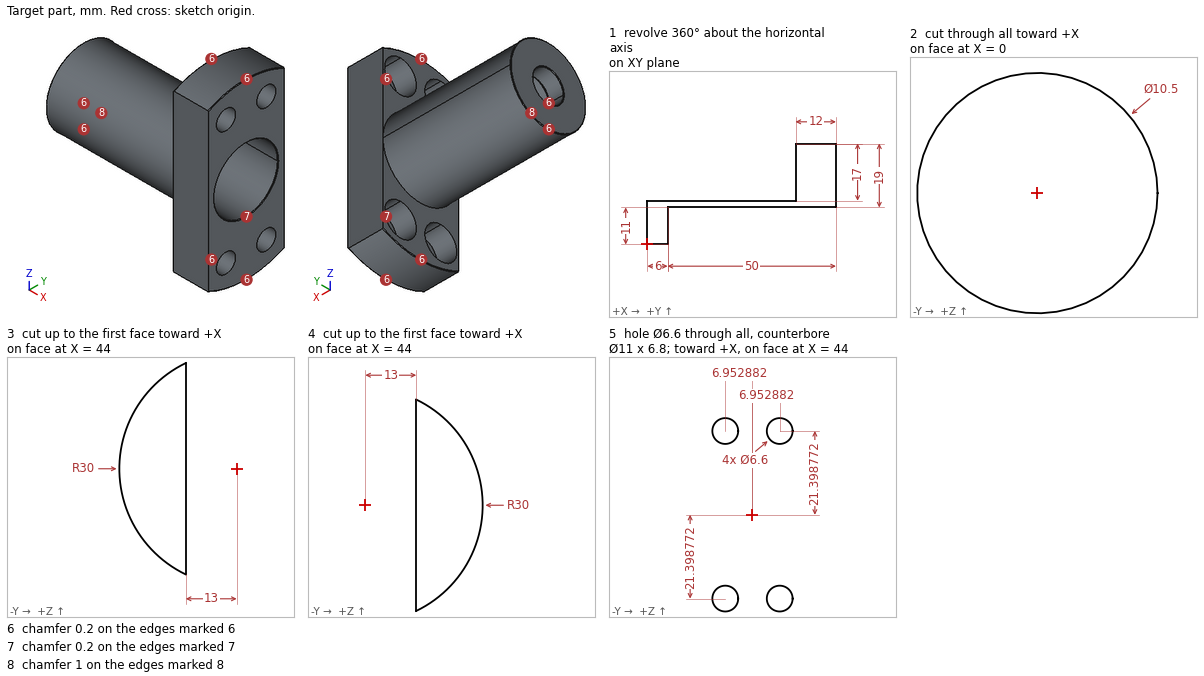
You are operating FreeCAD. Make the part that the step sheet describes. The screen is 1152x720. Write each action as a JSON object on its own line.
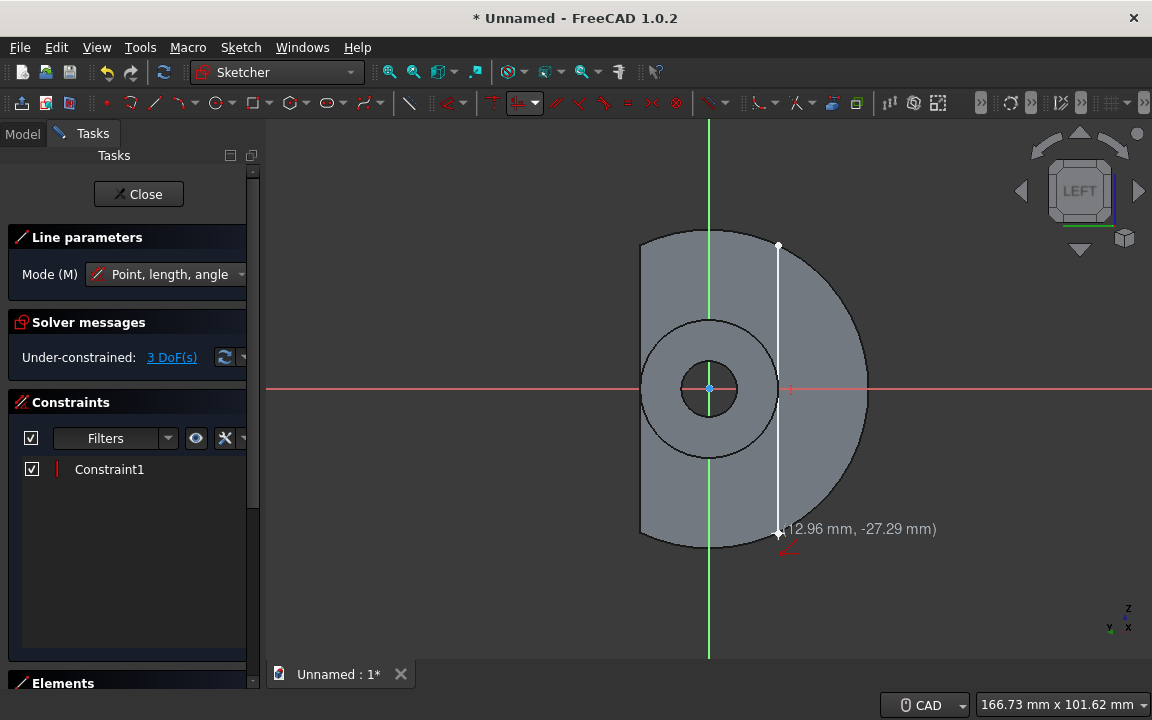
{"action": "left_click", "coordinate": [180, 104]}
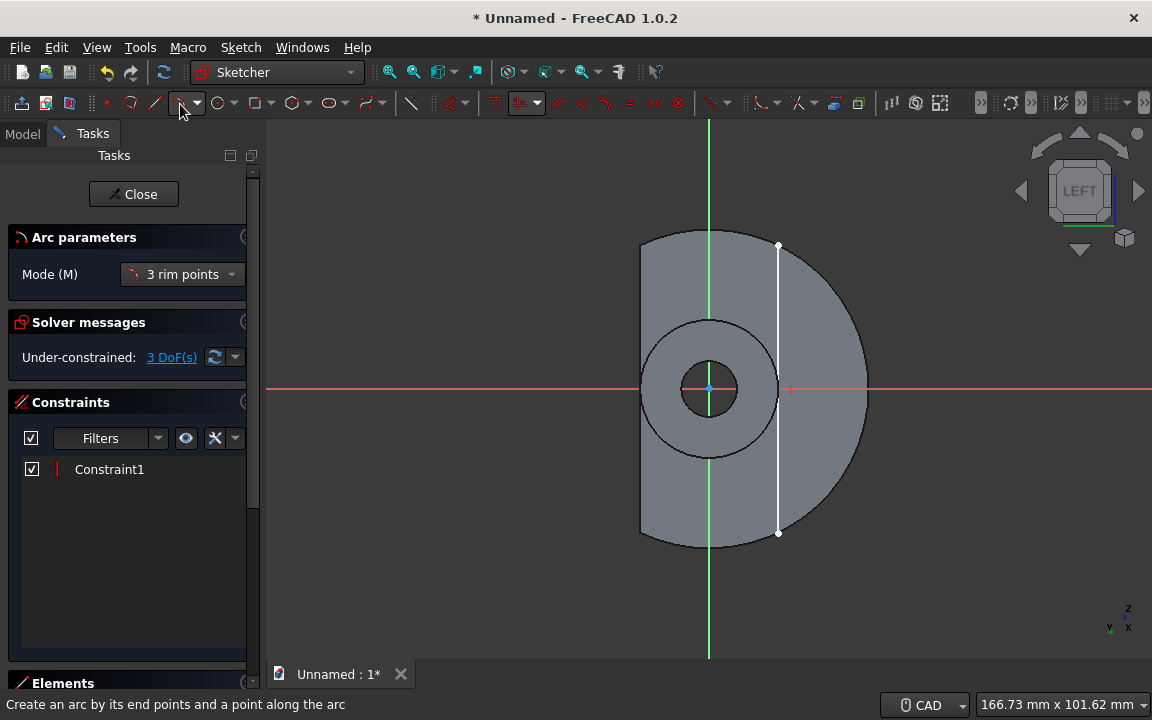
{"action": "left_click", "coordinate": [778, 534]}
{"action": "left_click", "coordinate": [778, 246]}
{"action": "left_click", "coordinate": [865, 424]}
{"action": "key", "text": "Escape"}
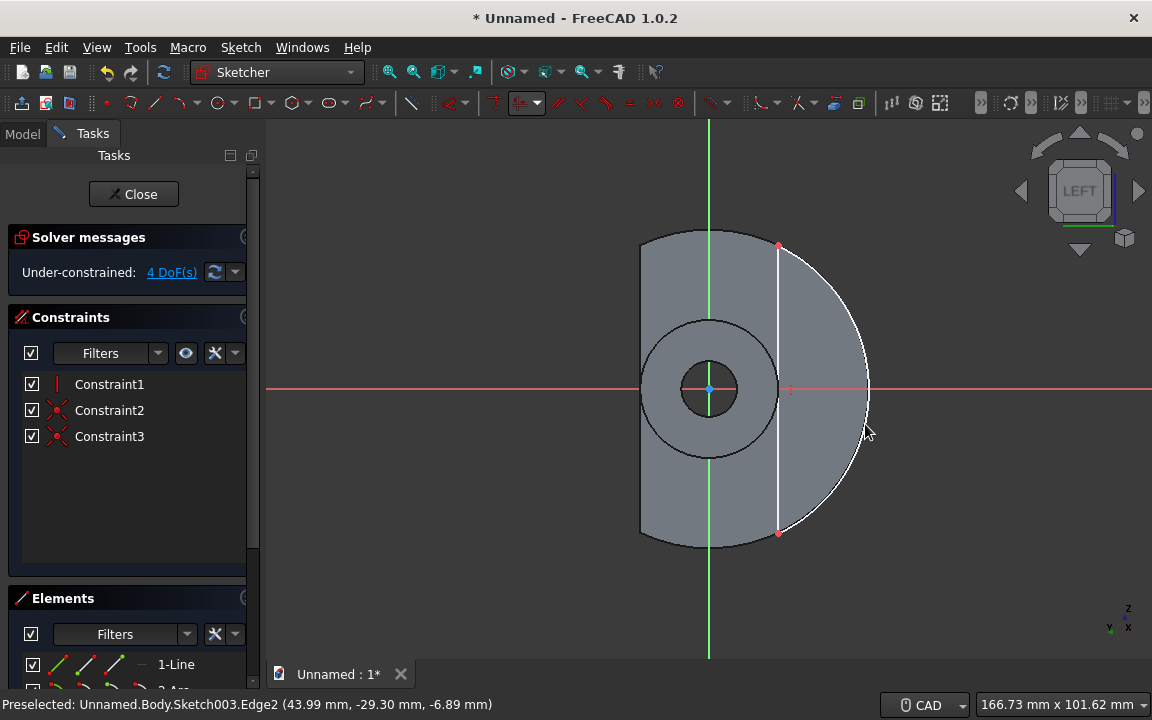
{"action": "left_click_drag", "start_coordinate": [699, 379], "coordinate": [719, 400]}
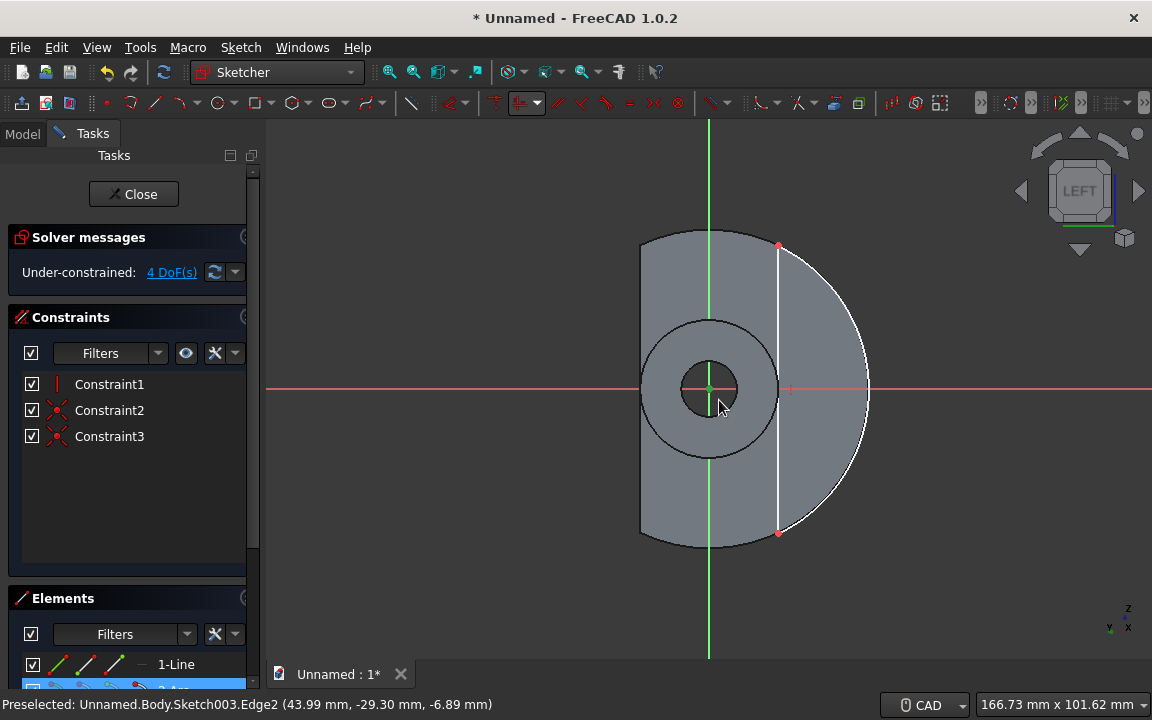
{"action": "key", "text": "c"}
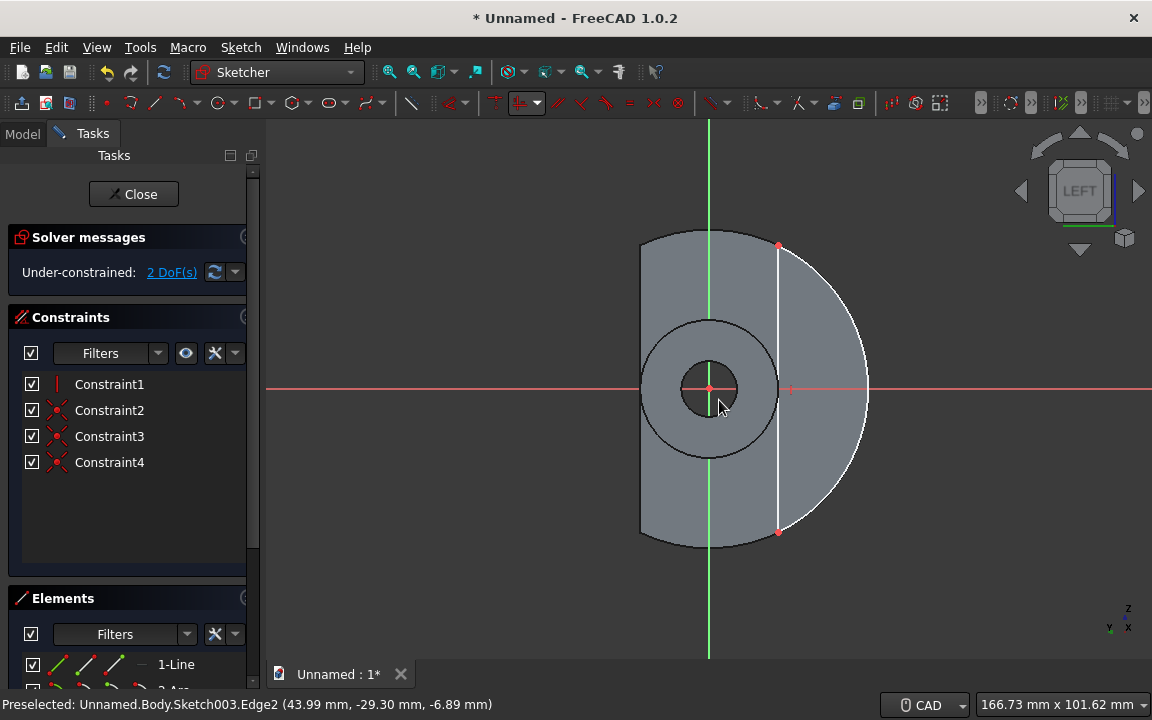
{"action": "left_click", "coordinate": [852, 458]}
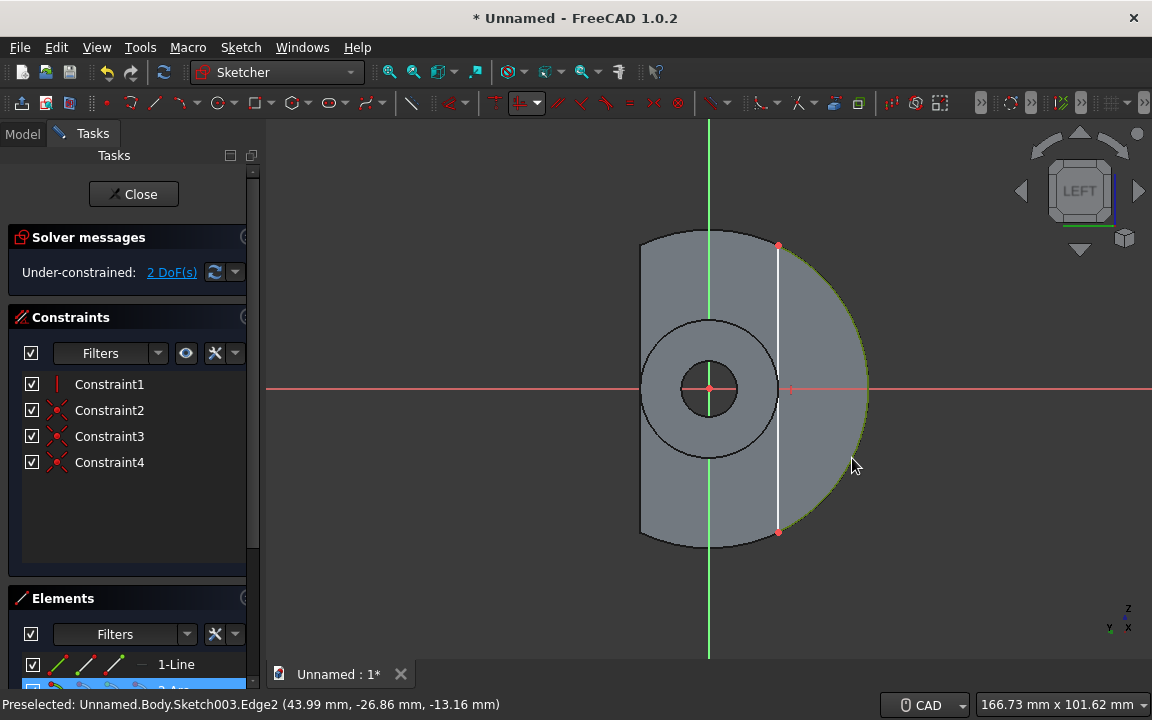
{"action": "key", "text": "k r"}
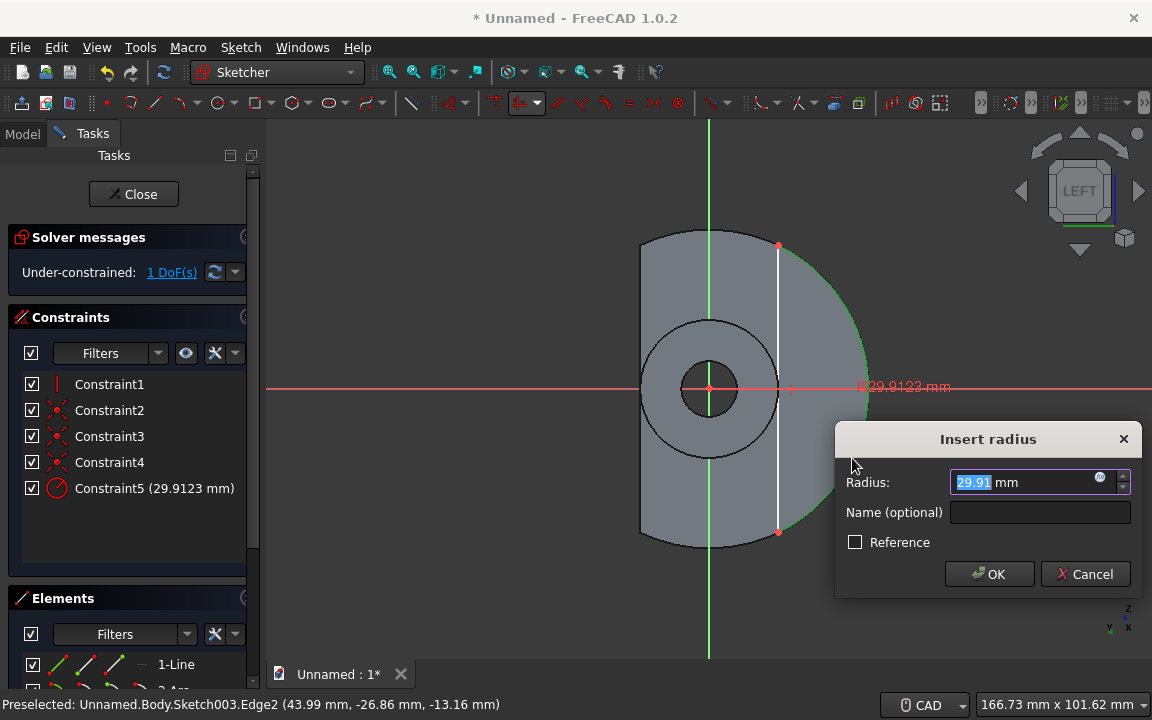
{"action": "type", "text": "30"}
{"action": "key", "text": "Return"}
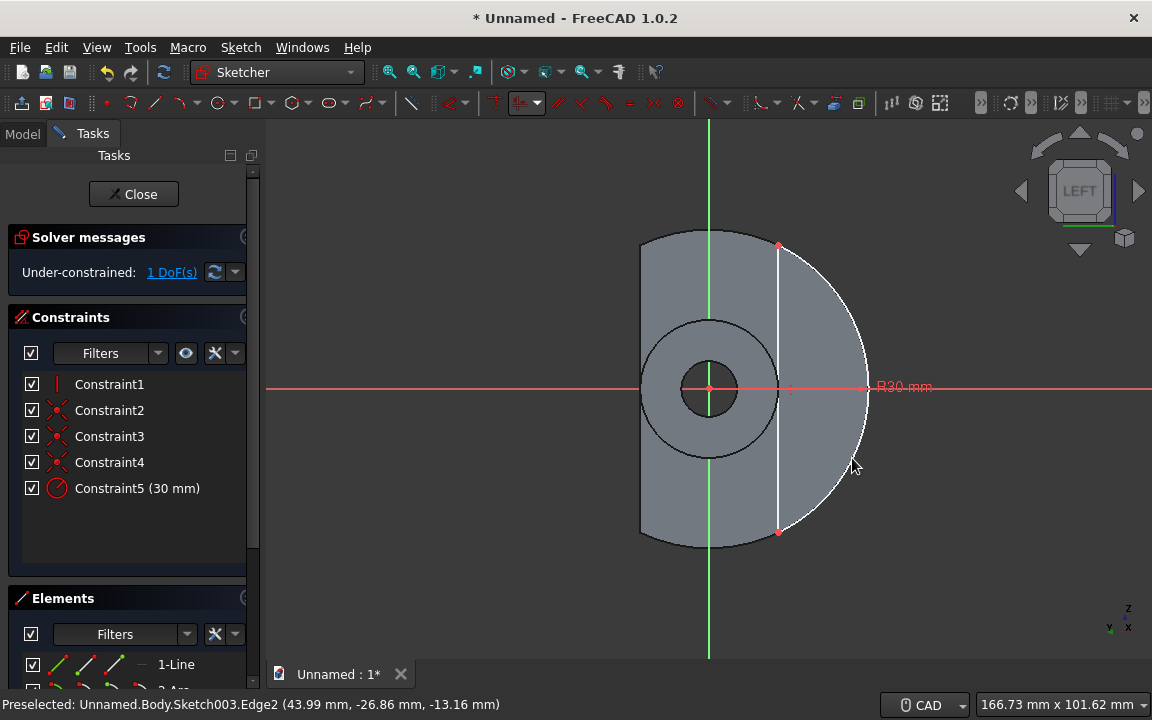
{"action": "left_click", "coordinate": [778, 245]}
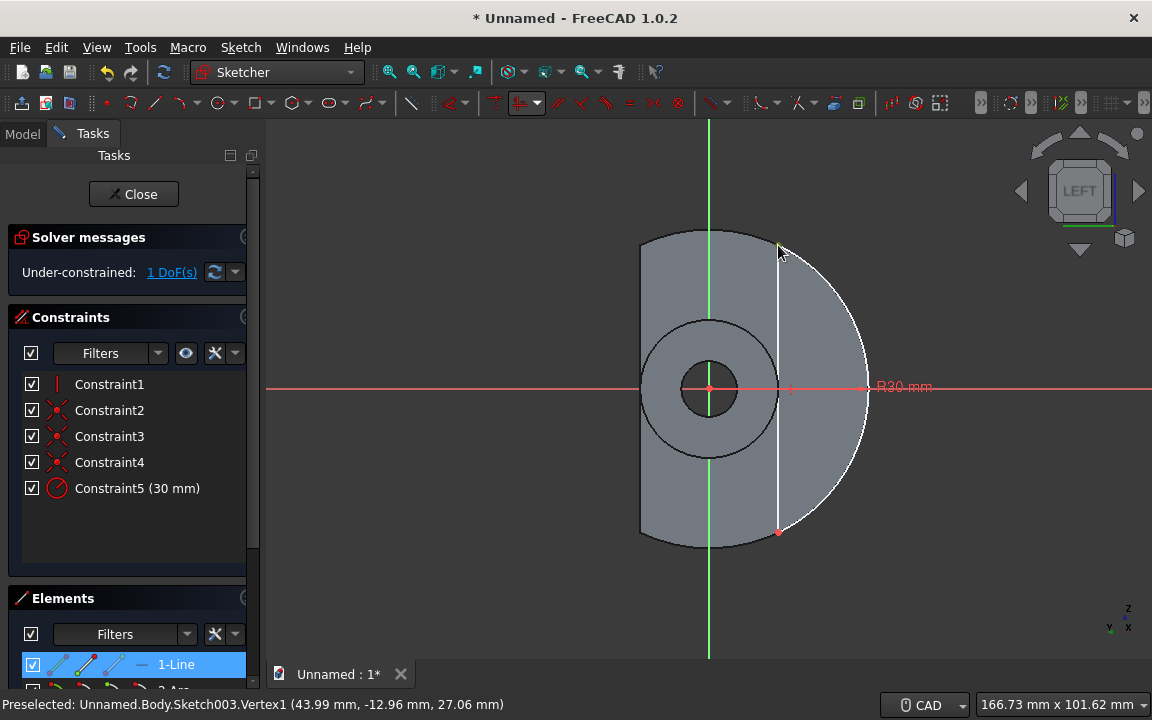
{"action": "left_click", "coordinate": [468, 104]}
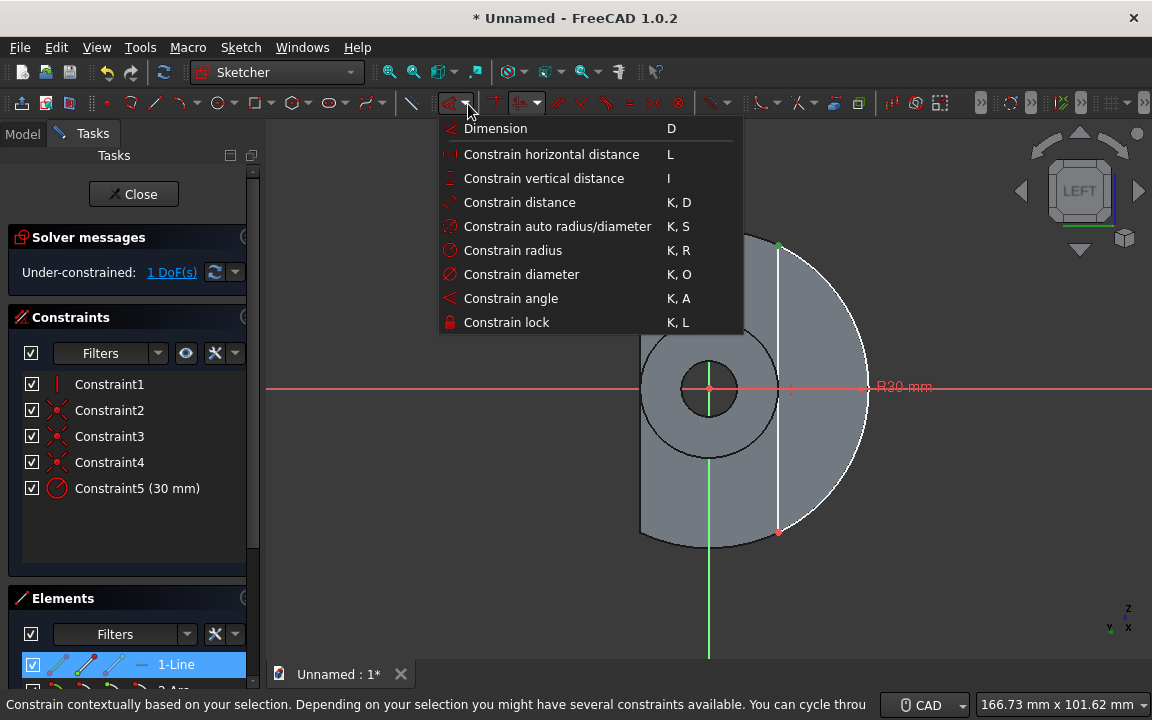
{"action": "left_click", "coordinate": [591, 154]}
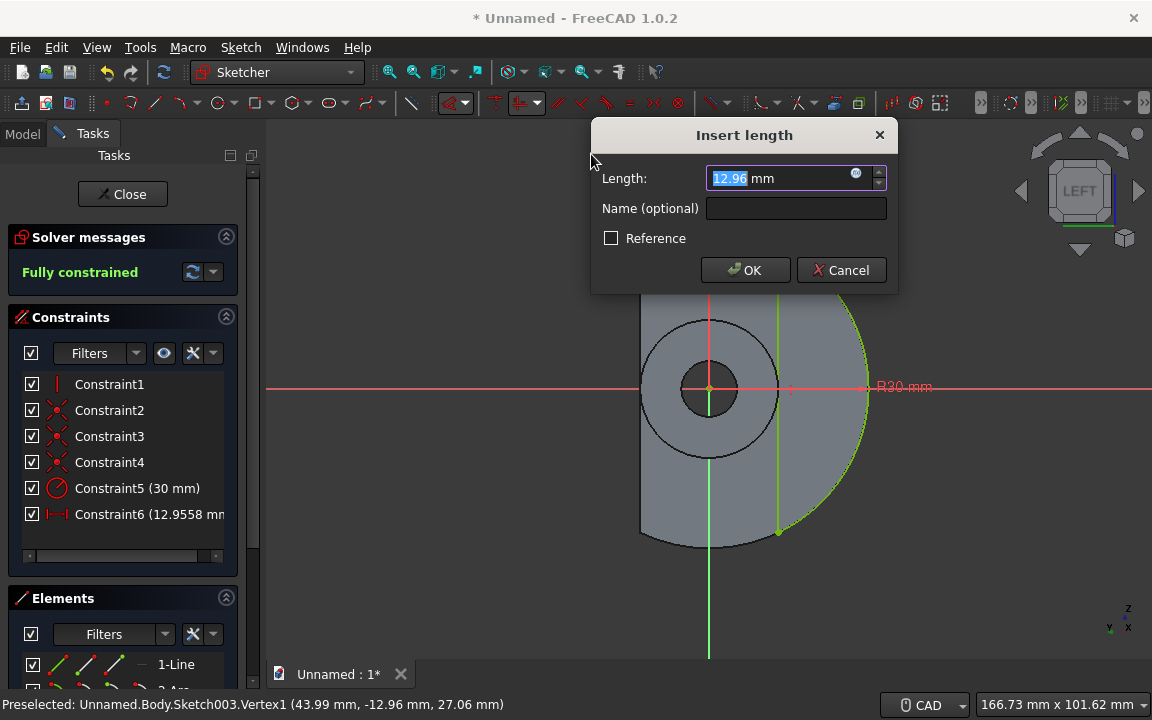
{"action": "type", "text": "13"}
{"action": "key", "text": "Return"}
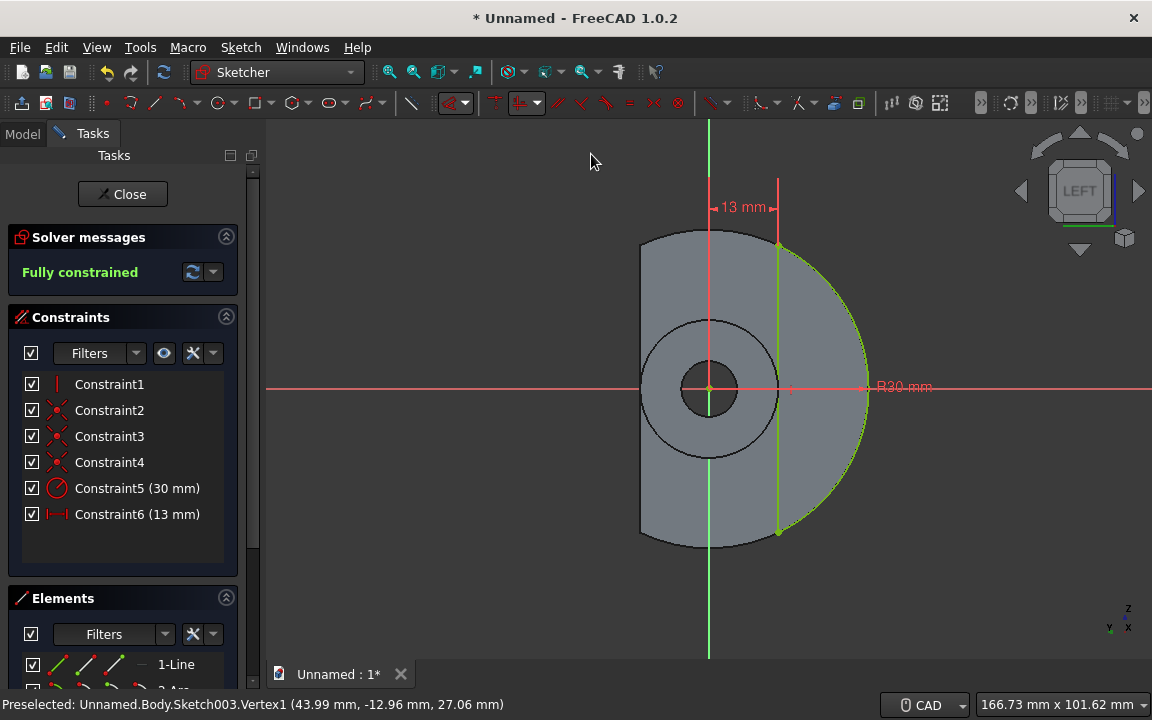
{"action": "left_click", "coordinate": [123, 194]}